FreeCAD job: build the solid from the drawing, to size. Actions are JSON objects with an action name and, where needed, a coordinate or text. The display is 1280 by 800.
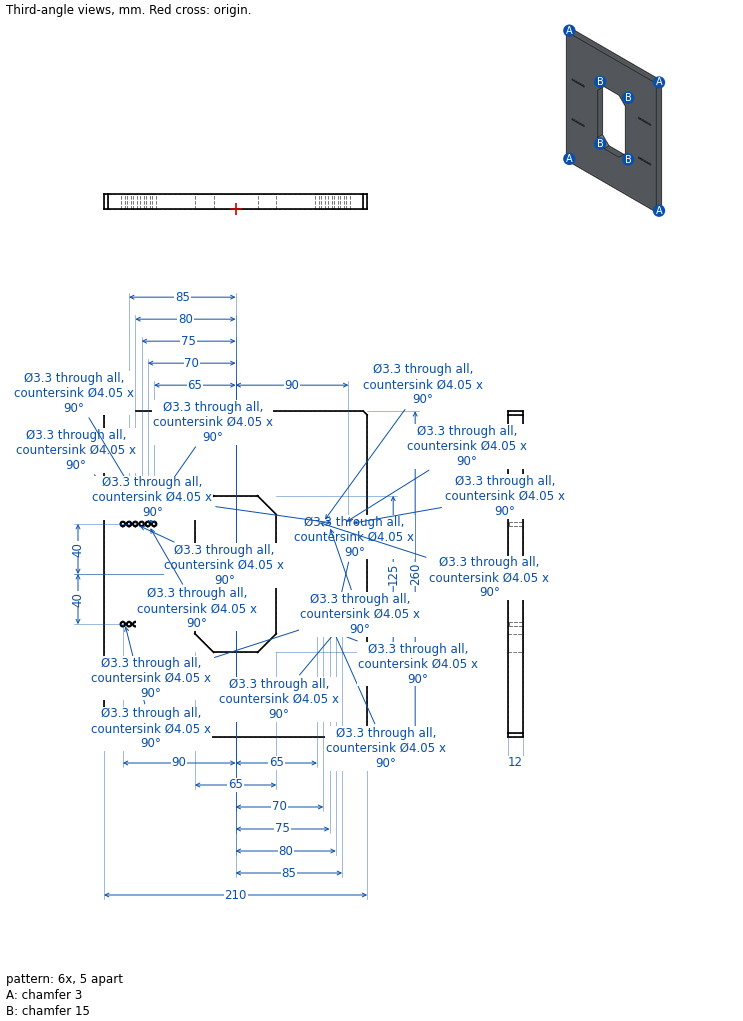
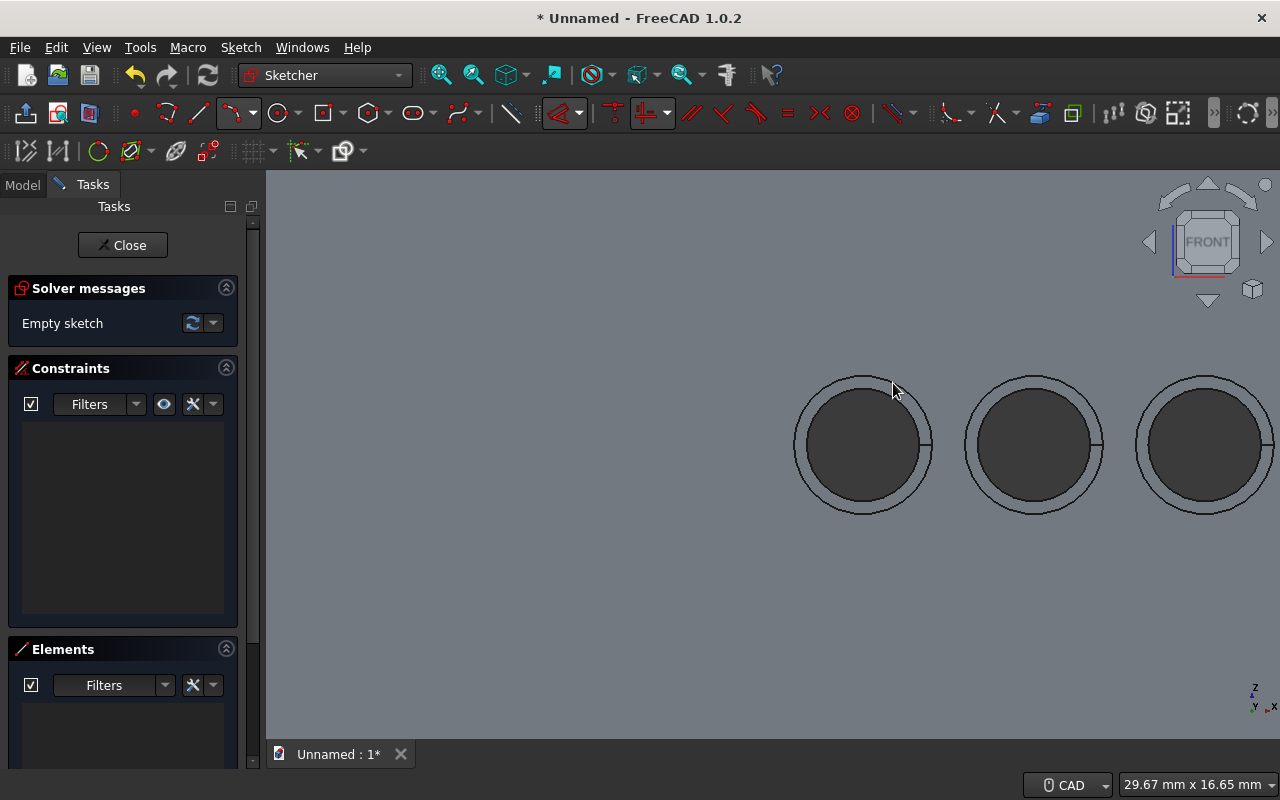
{"action": "scroll", "coordinate": [687, 441], "scroll_direction": "up", "scroll_amount": 6}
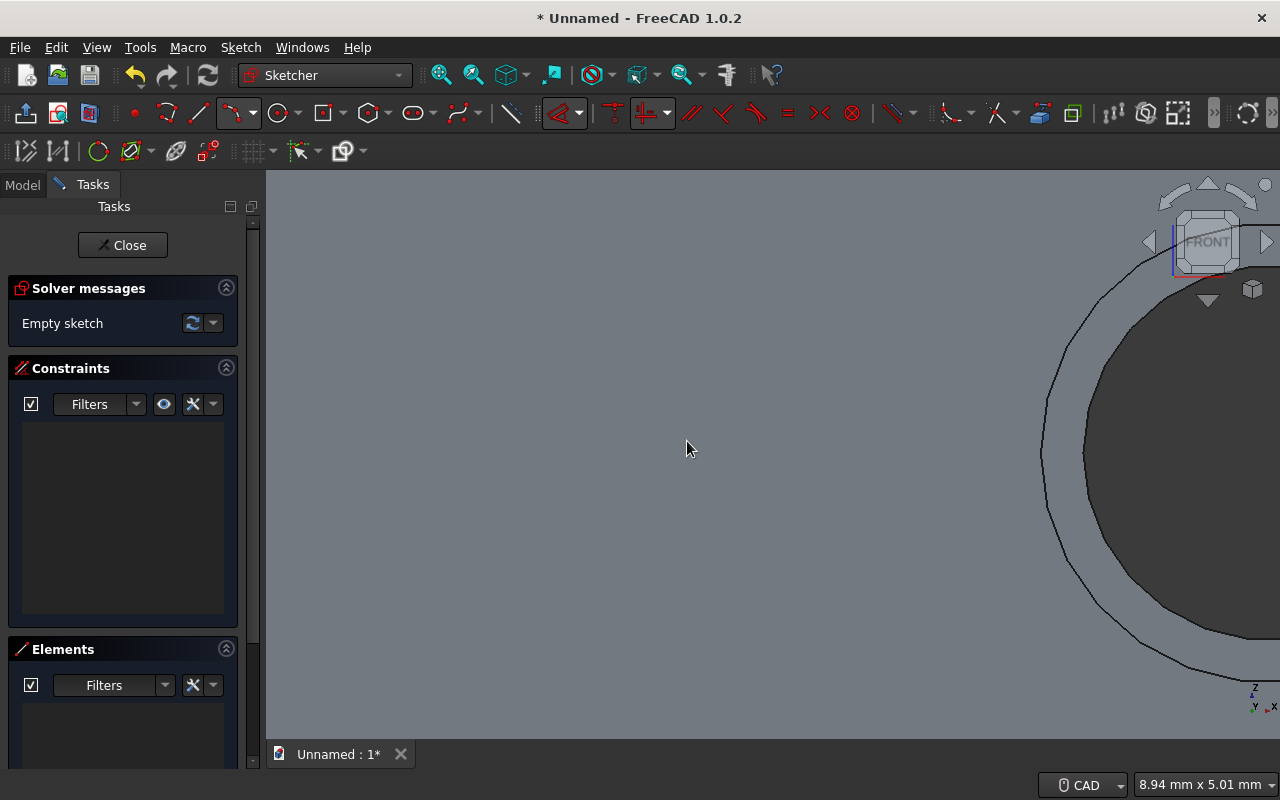
{"action": "left_click", "coordinate": [278, 114]}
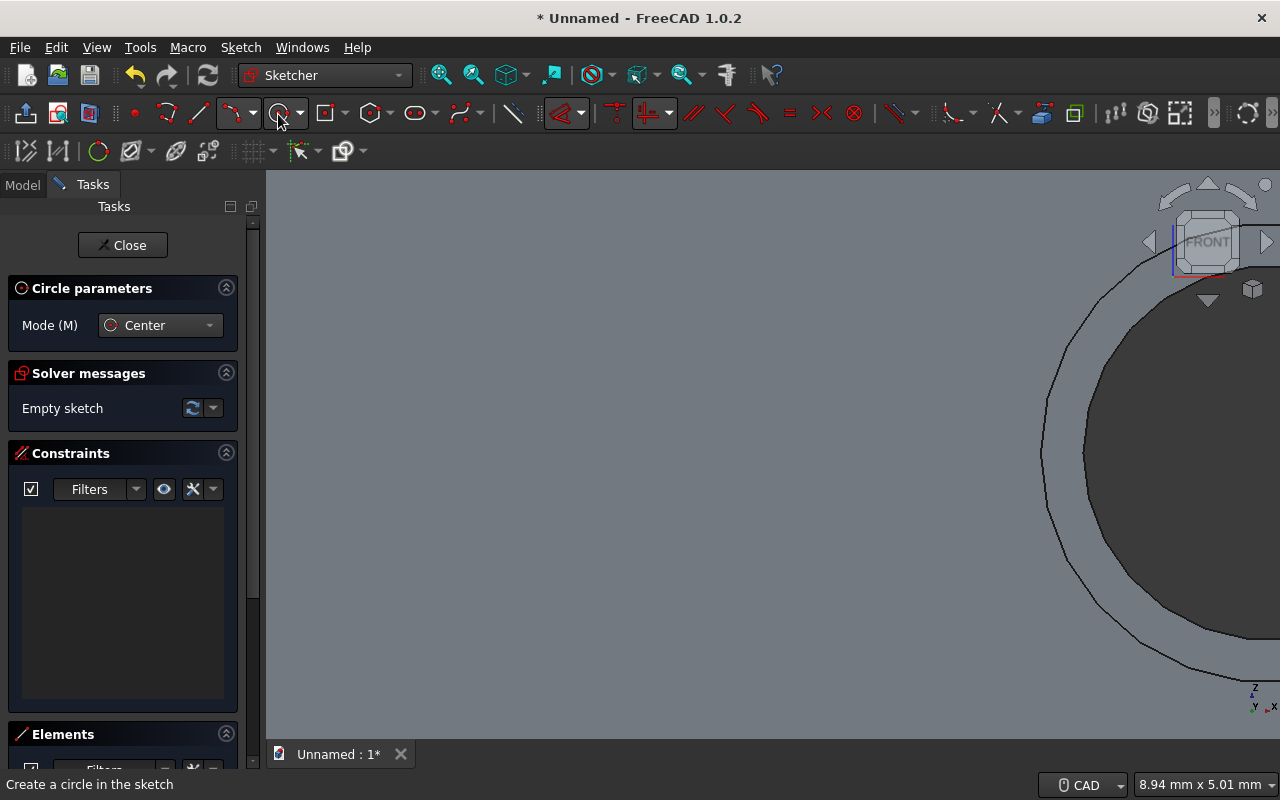
{"action": "left_click", "coordinate": [703, 453]}
{"action": "mouse_move", "coordinate": [836, 321]}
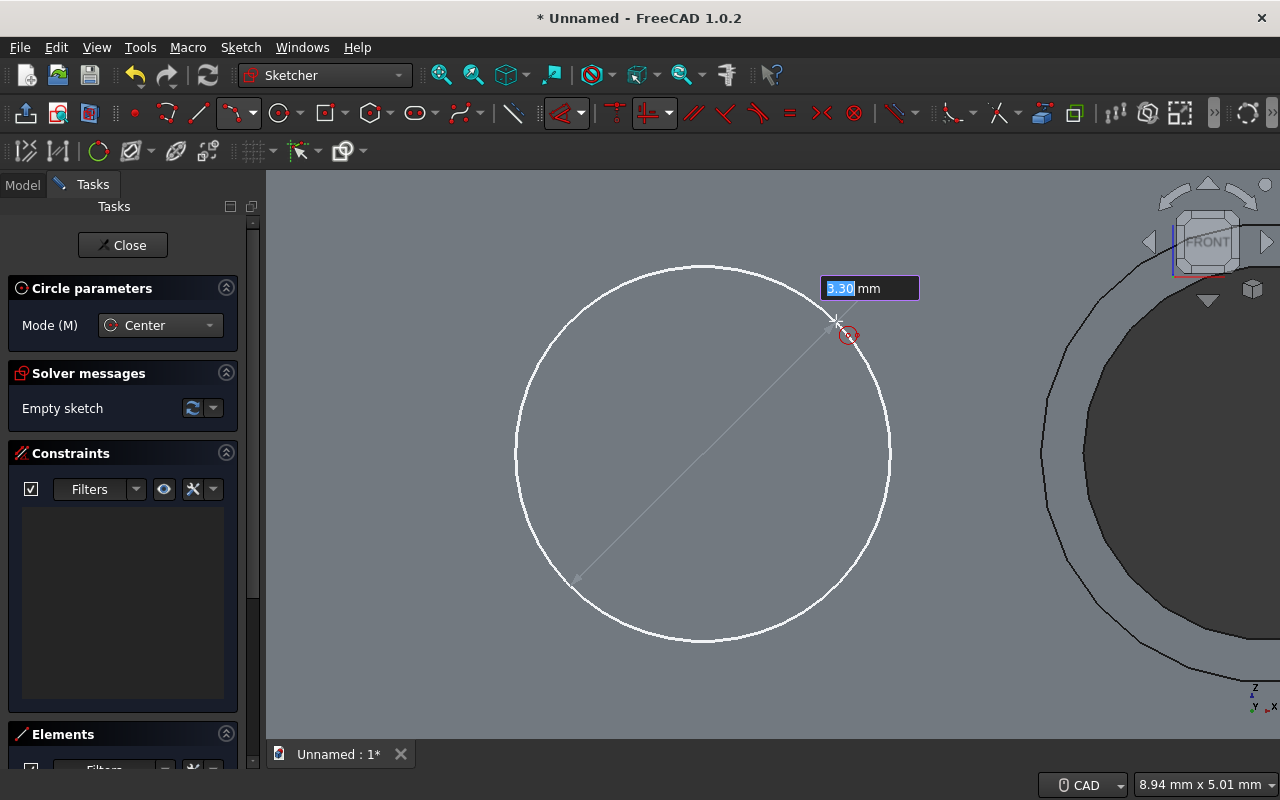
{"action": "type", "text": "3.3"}
{"action": "key", "text": "Return"}
{"action": "key", "text": "Escape"}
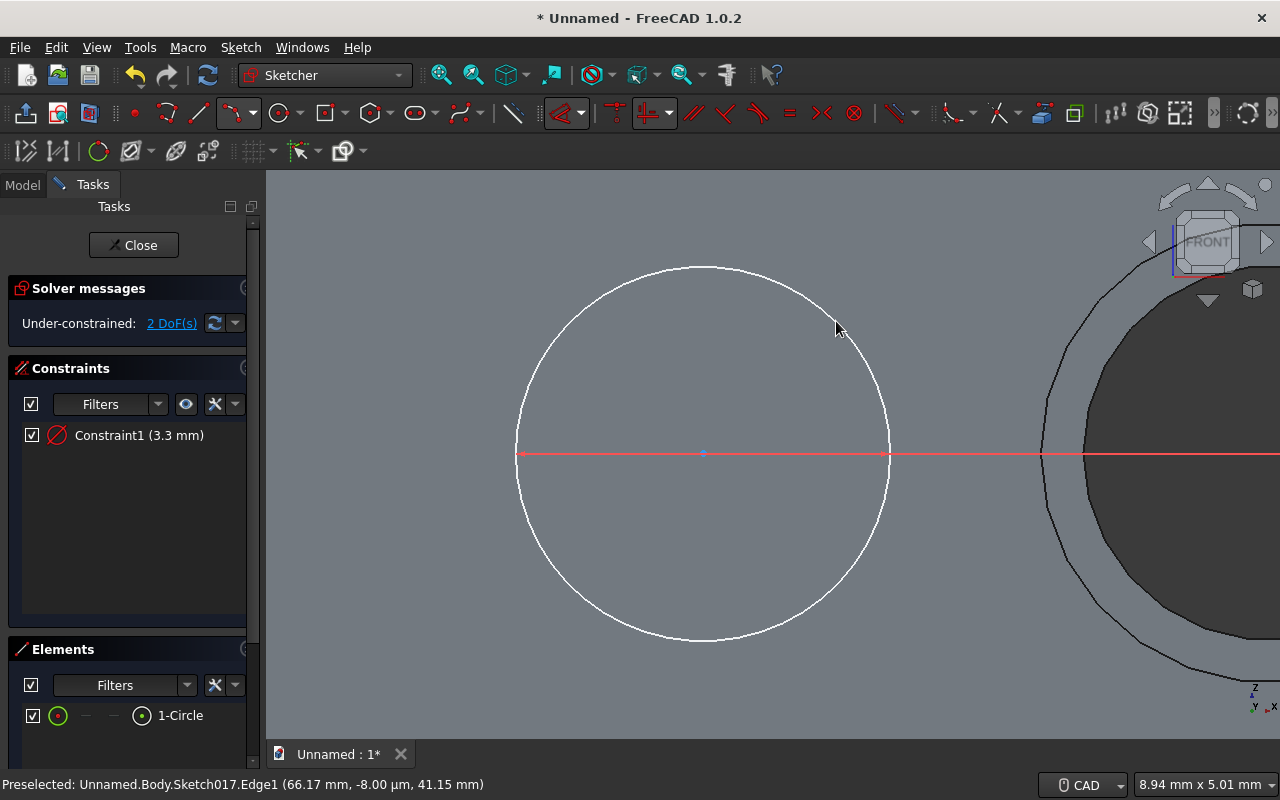
{"action": "left_click", "coordinate": [703, 454]}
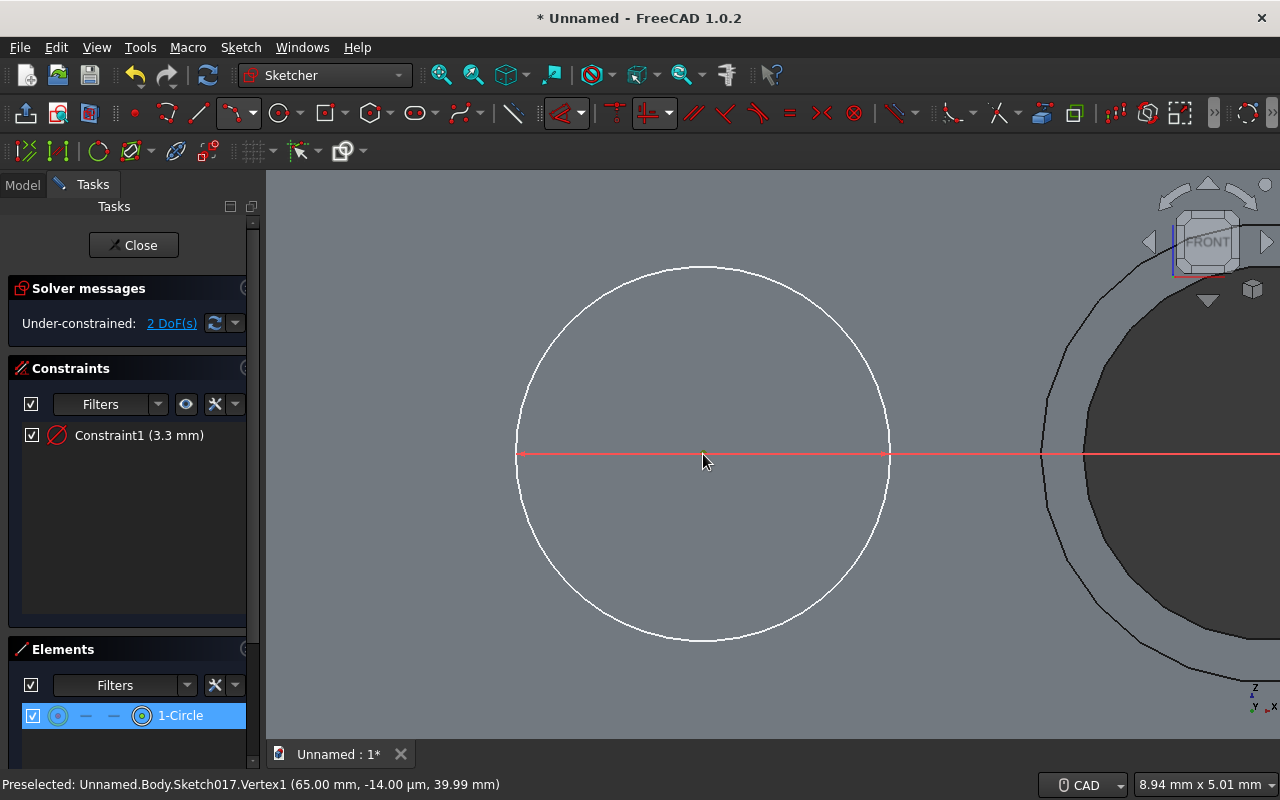
{"action": "left_click", "coordinate": [584, 114]}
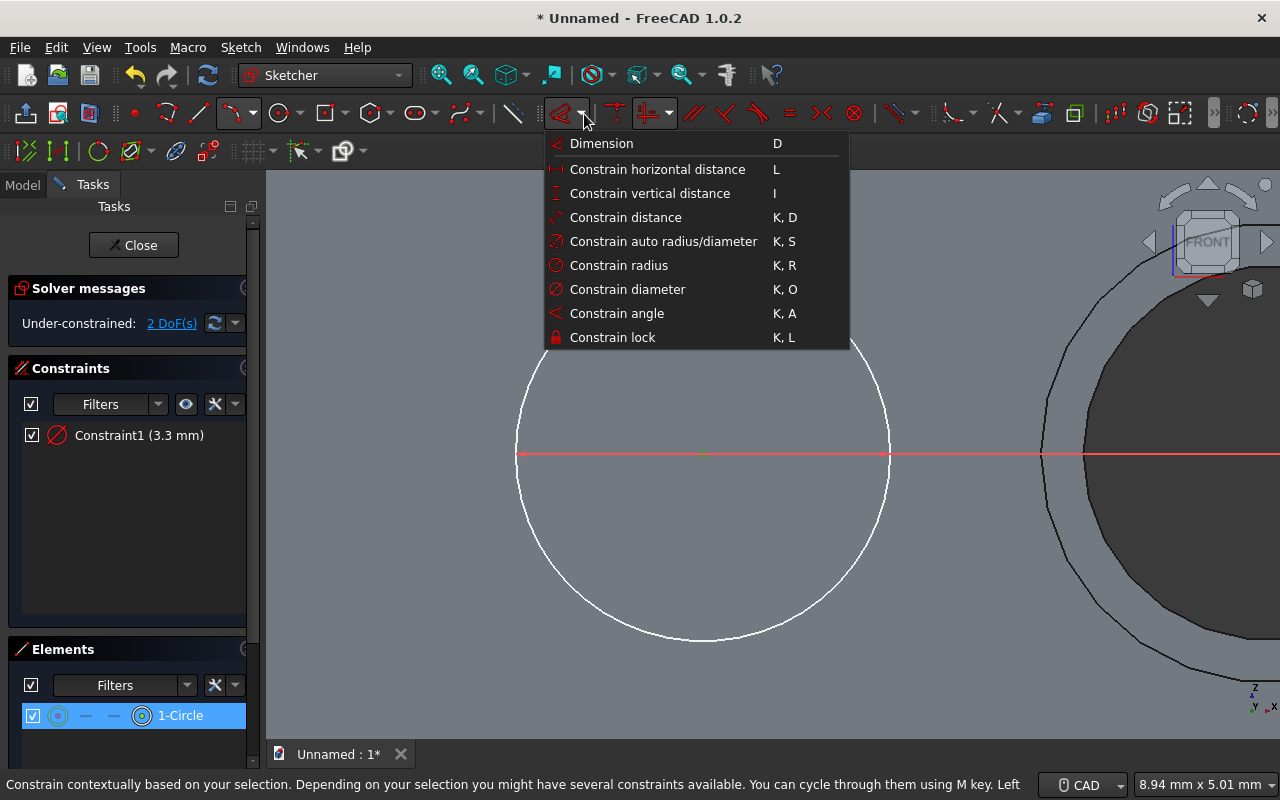
{"action": "left_click", "coordinate": [697, 169]}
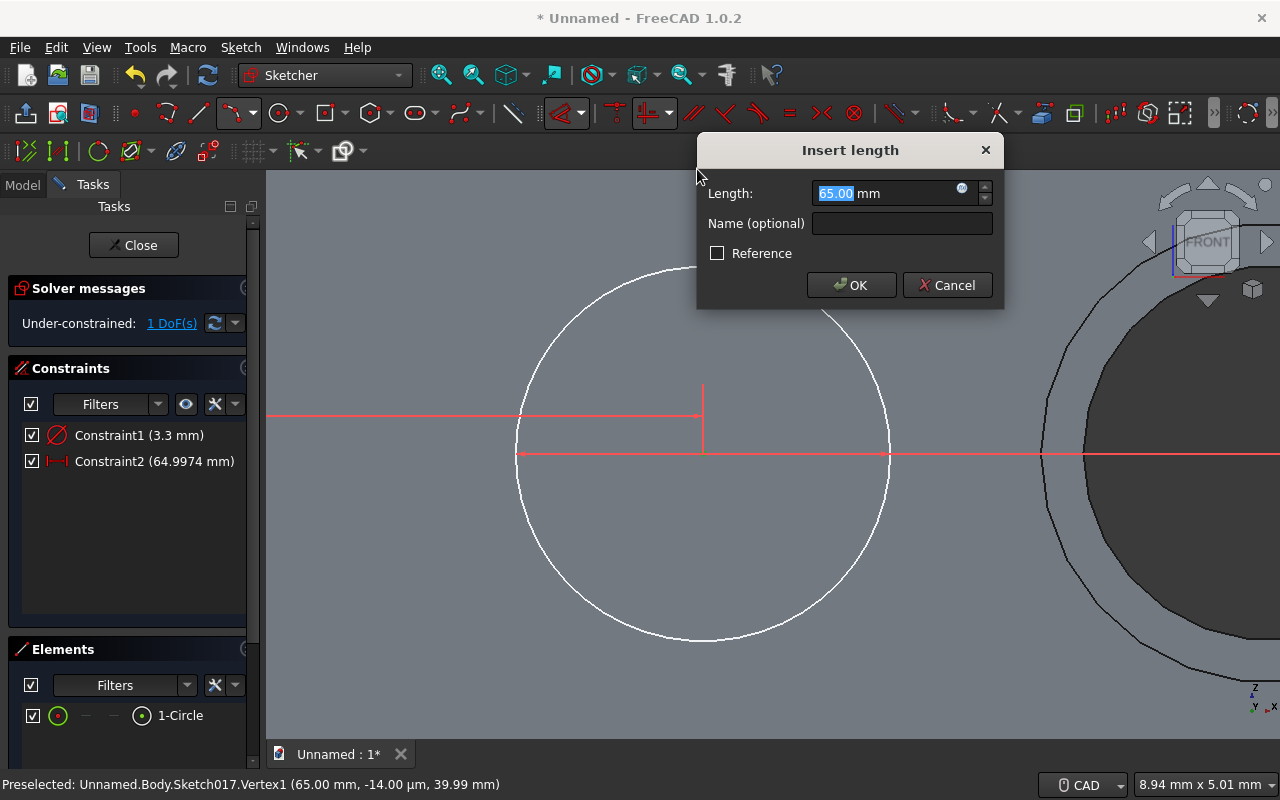
{"action": "type", "text": "65"}
{"action": "key", "text": "Return"}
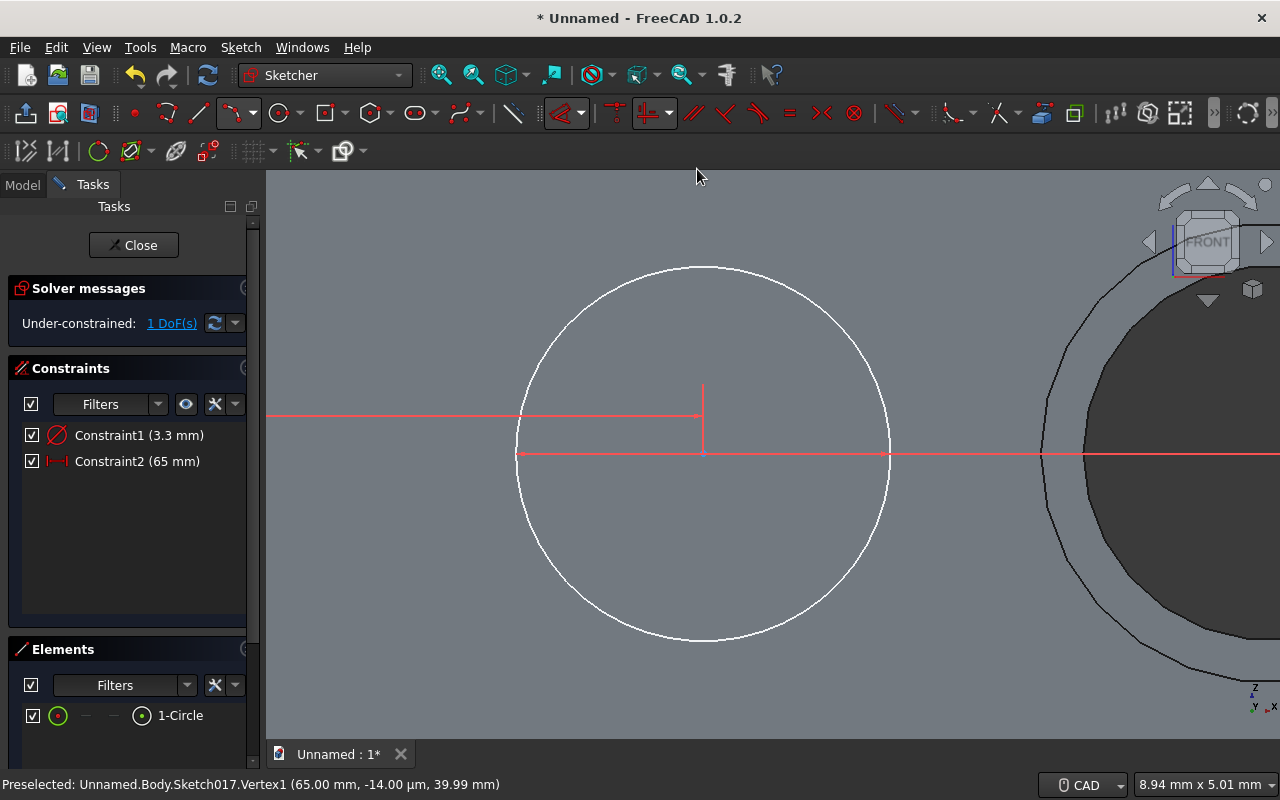
{"action": "left_click", "coordinate": [703, 454]}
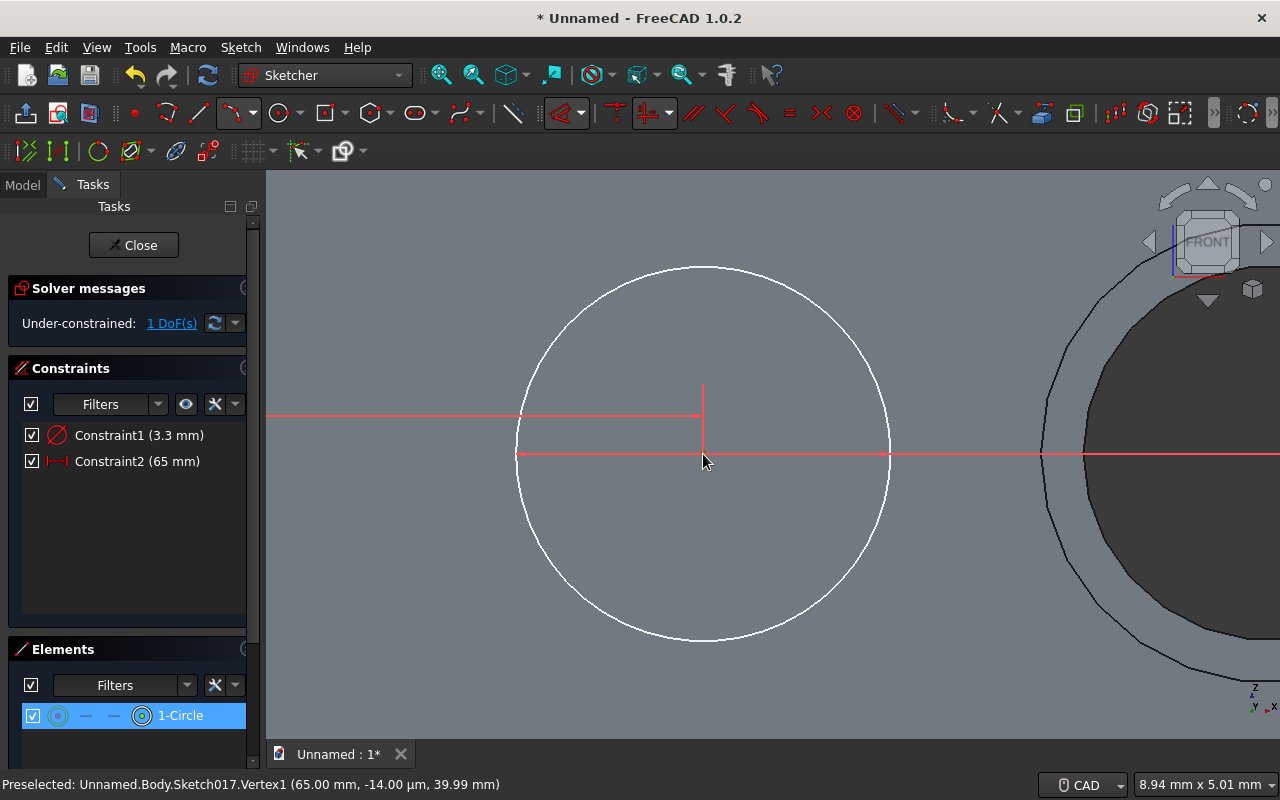
{"action": "left_click", "coordinate": [584, 114]}